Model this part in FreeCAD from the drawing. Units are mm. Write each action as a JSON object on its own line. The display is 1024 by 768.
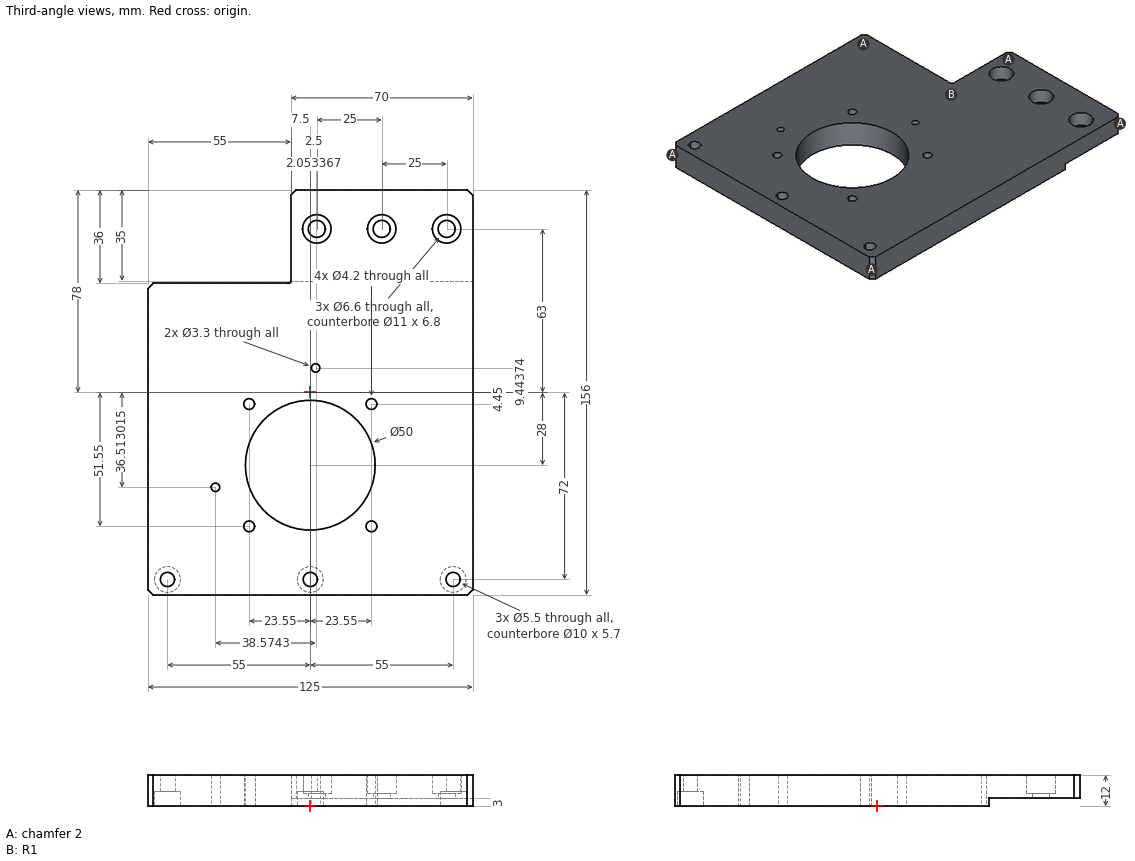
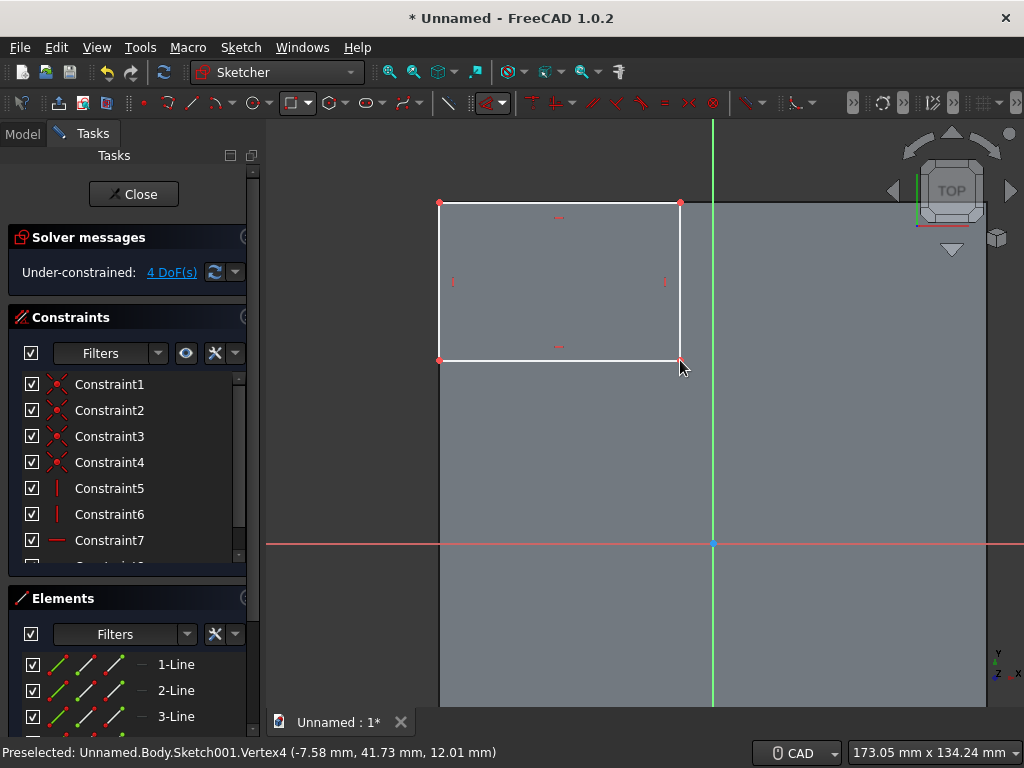
{"action": "left_click", "coordinate": [439, 250]}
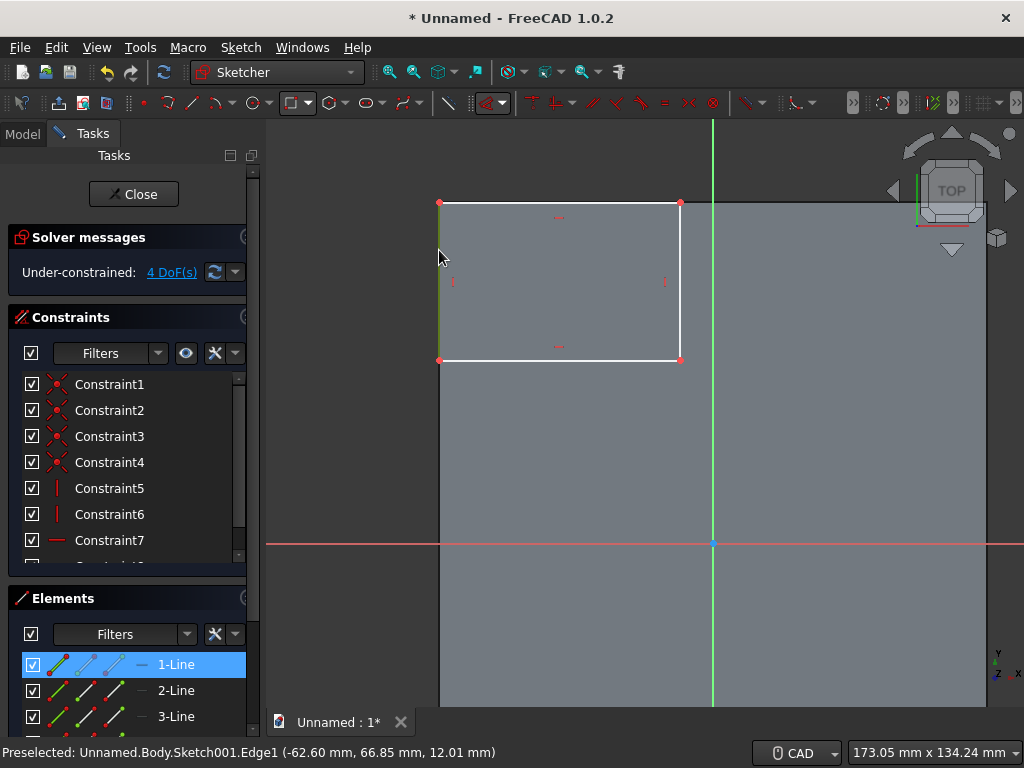
{"action": "key", "text": "i"}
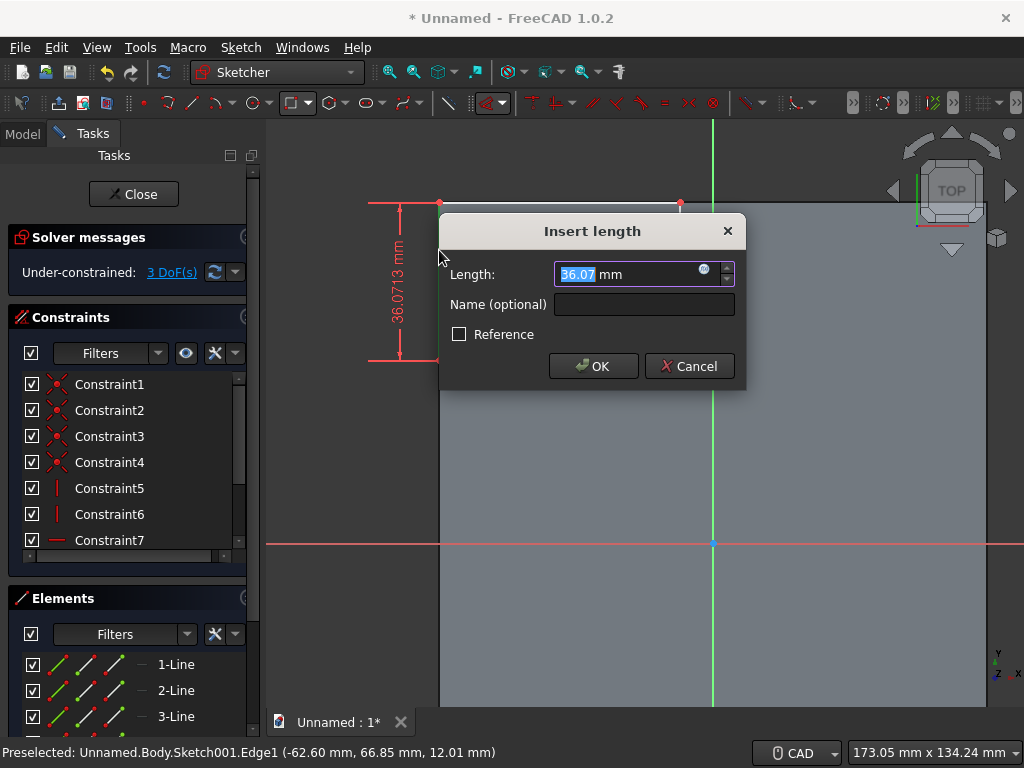
{"action": "type", "text": "36"}
{"action": "key", "text": "Return"}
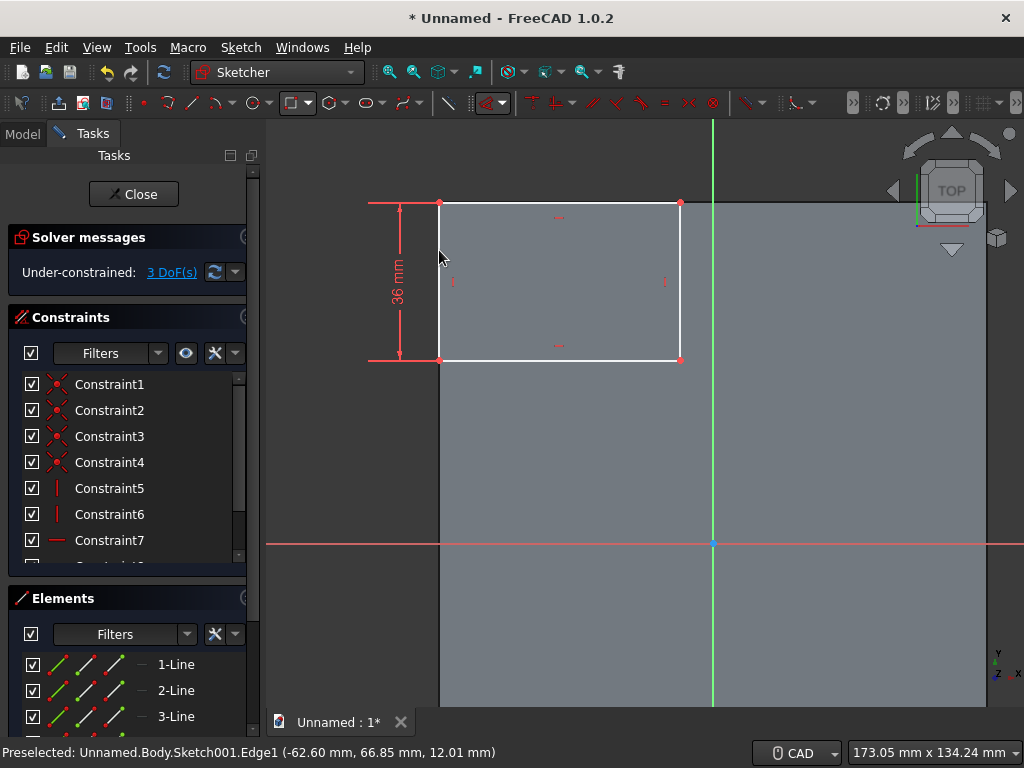
{"action": "left_click", "coordinate": [511, 361]}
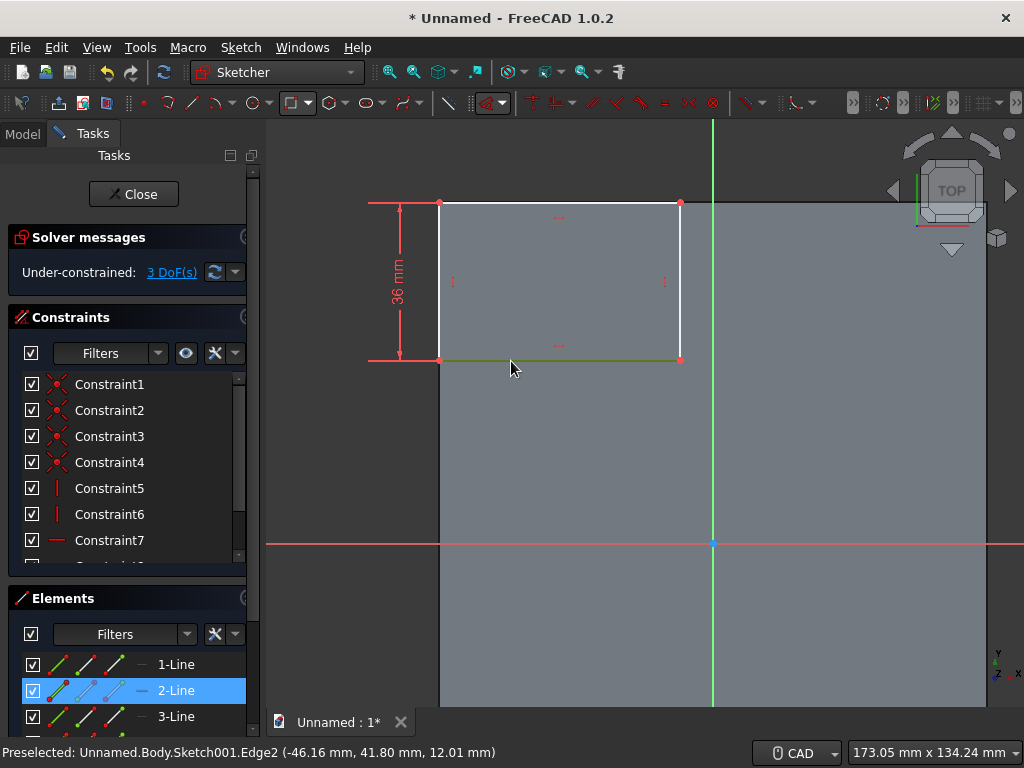
{"action": "key", "text": "l"}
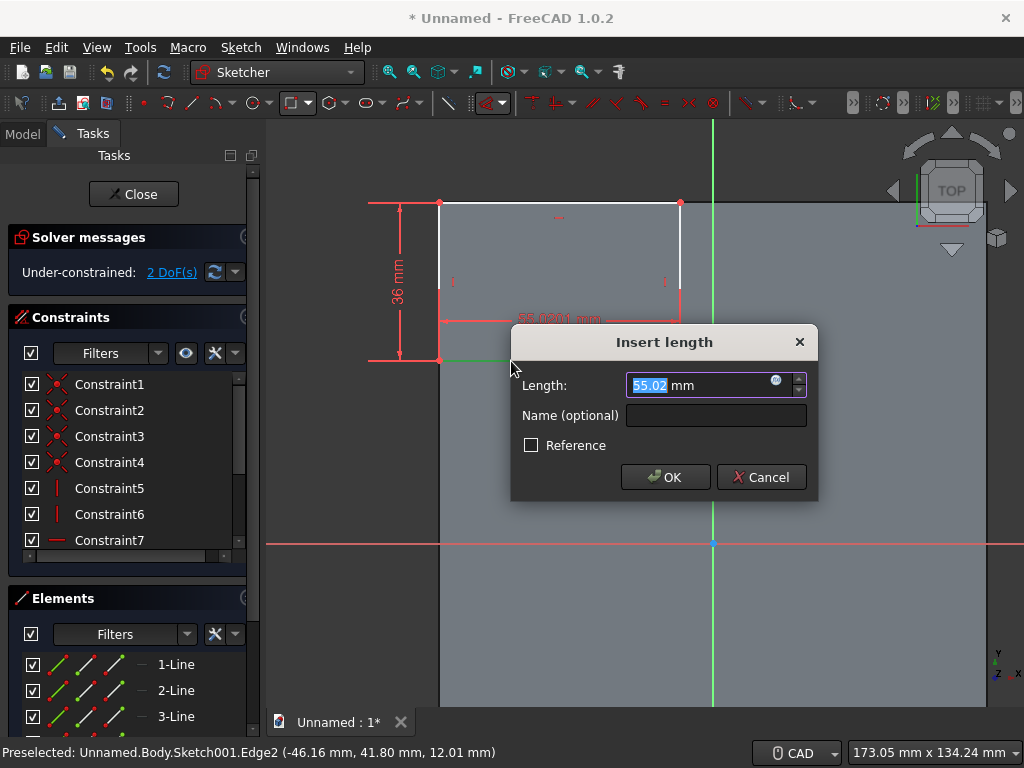
{"action": "type", "text": "55"}
{"action": "key", "text": "Return"}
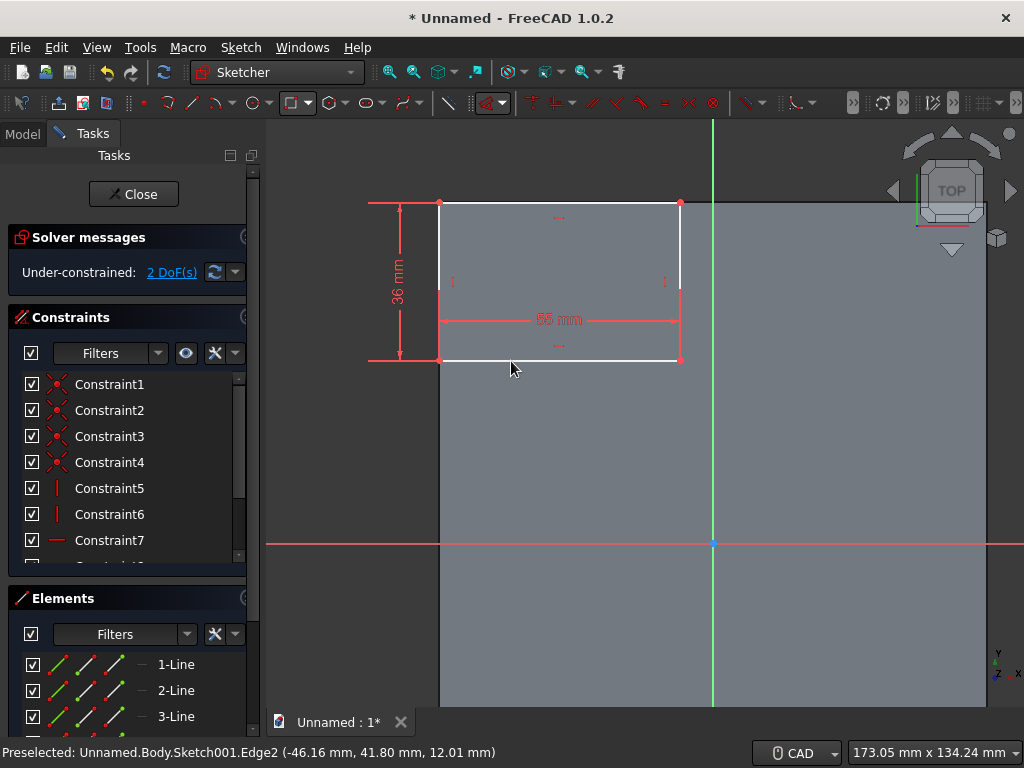
{"action": "left_click", "coordinate": [439, 203]}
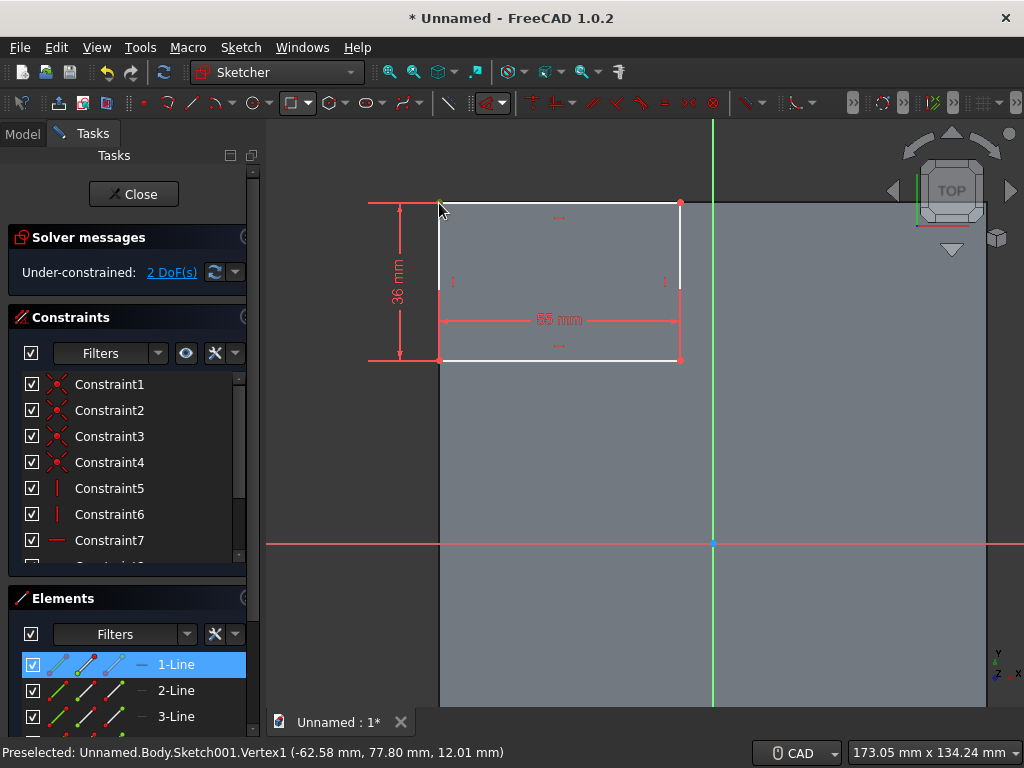
{"action": "left_click", "coordinate": [504, 104]}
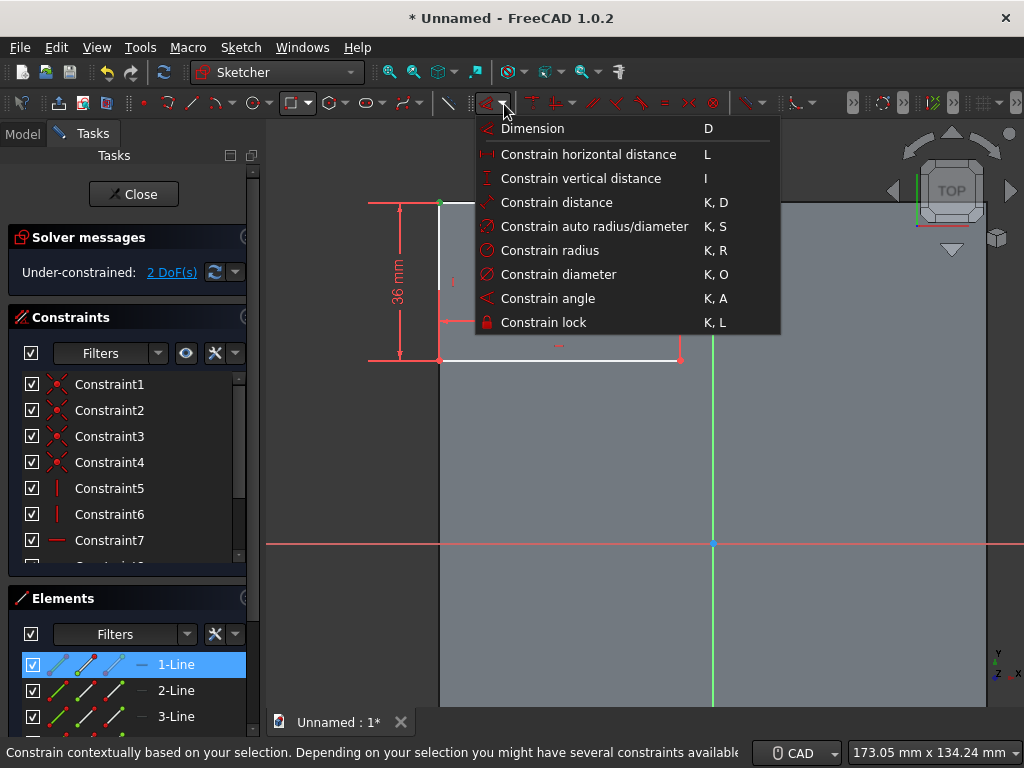
{"action": "left_click", "coordinate": [628, 178]}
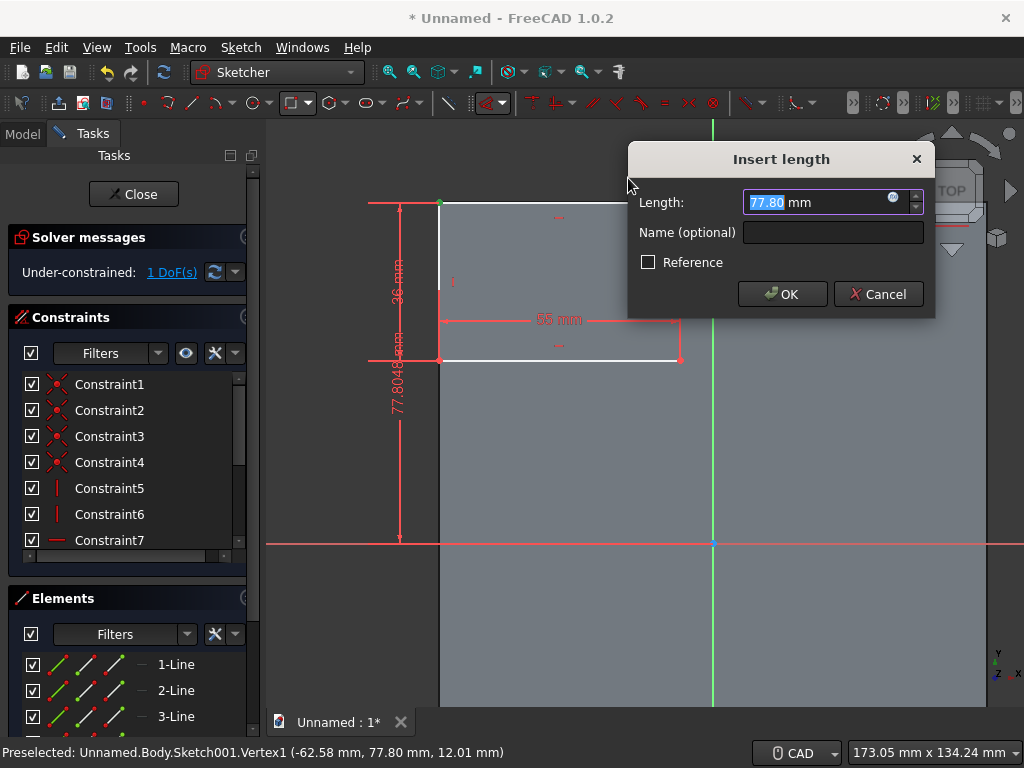
{"action": "type", "text": "78"}
{"action": "key", "text": "Return"}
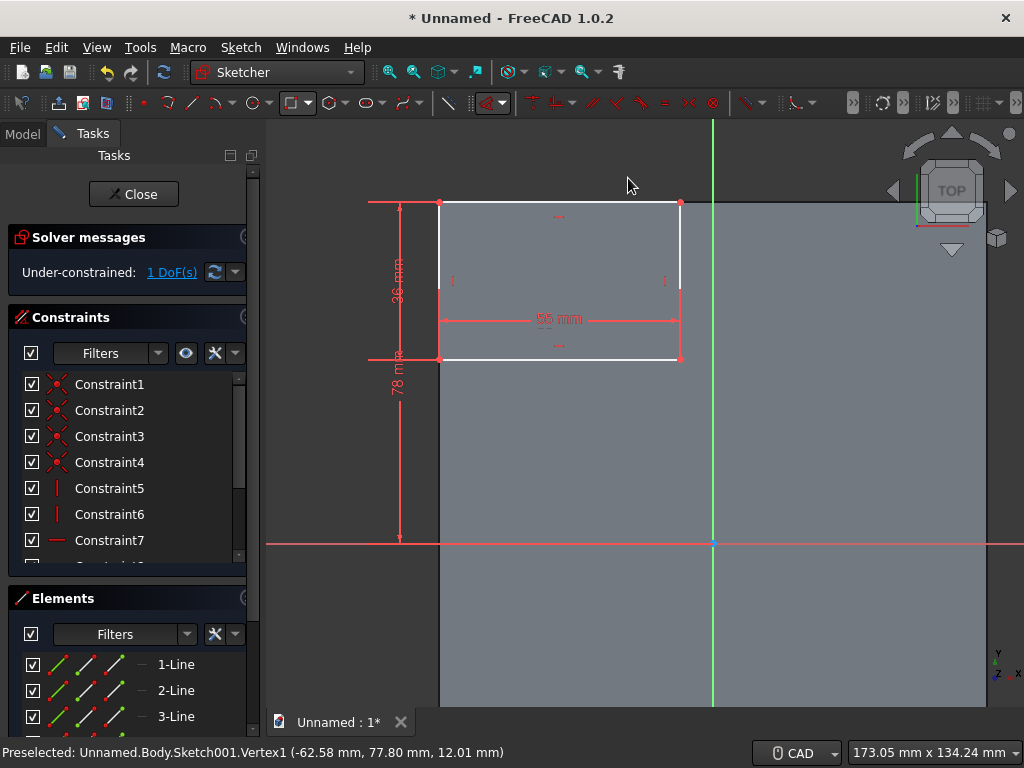
{"action": "left_click", "coordinate": [680, 360]}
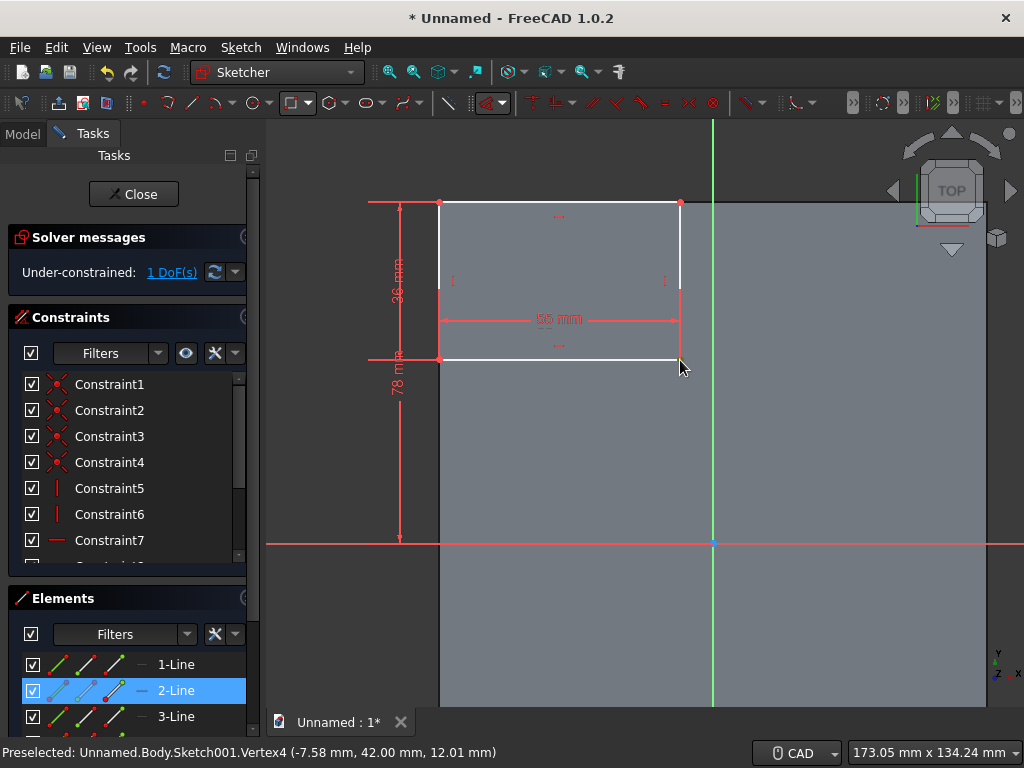
{"action": "left_click", "coordinate": [504, 104]}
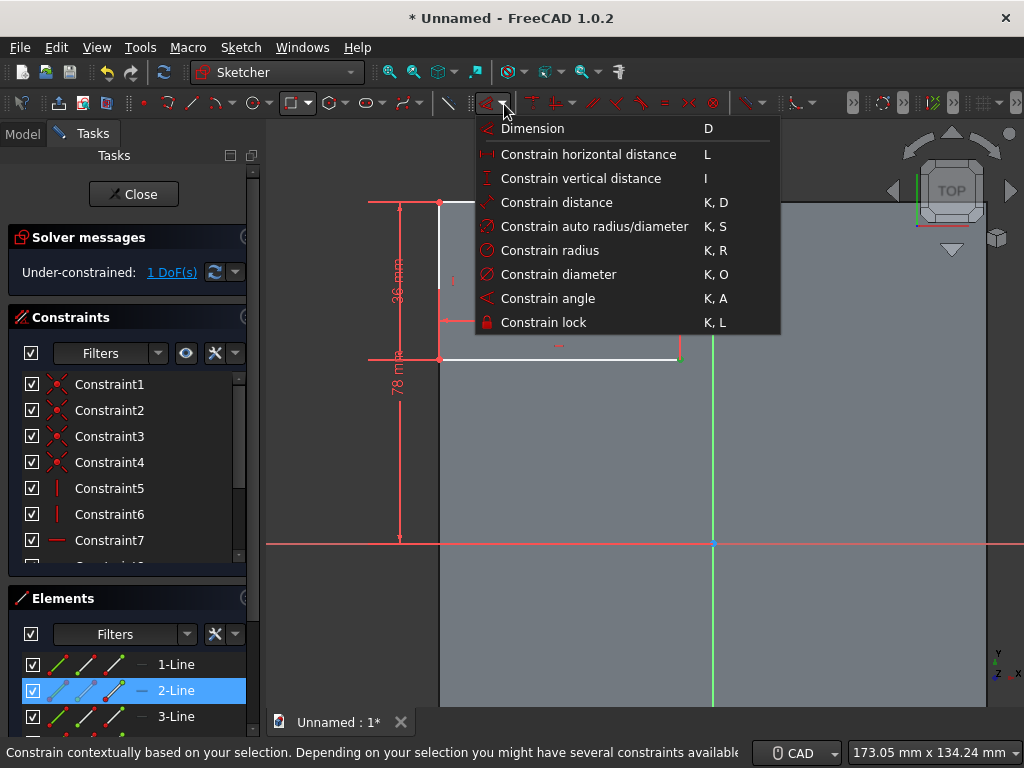
{"action": "left_click", "coordinate": [628, 154]}